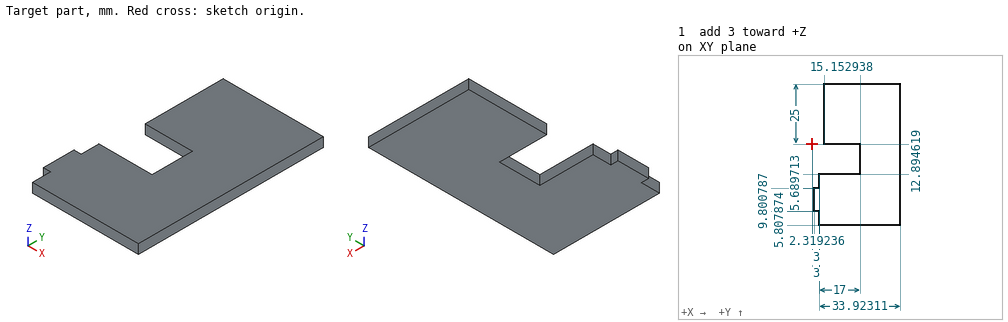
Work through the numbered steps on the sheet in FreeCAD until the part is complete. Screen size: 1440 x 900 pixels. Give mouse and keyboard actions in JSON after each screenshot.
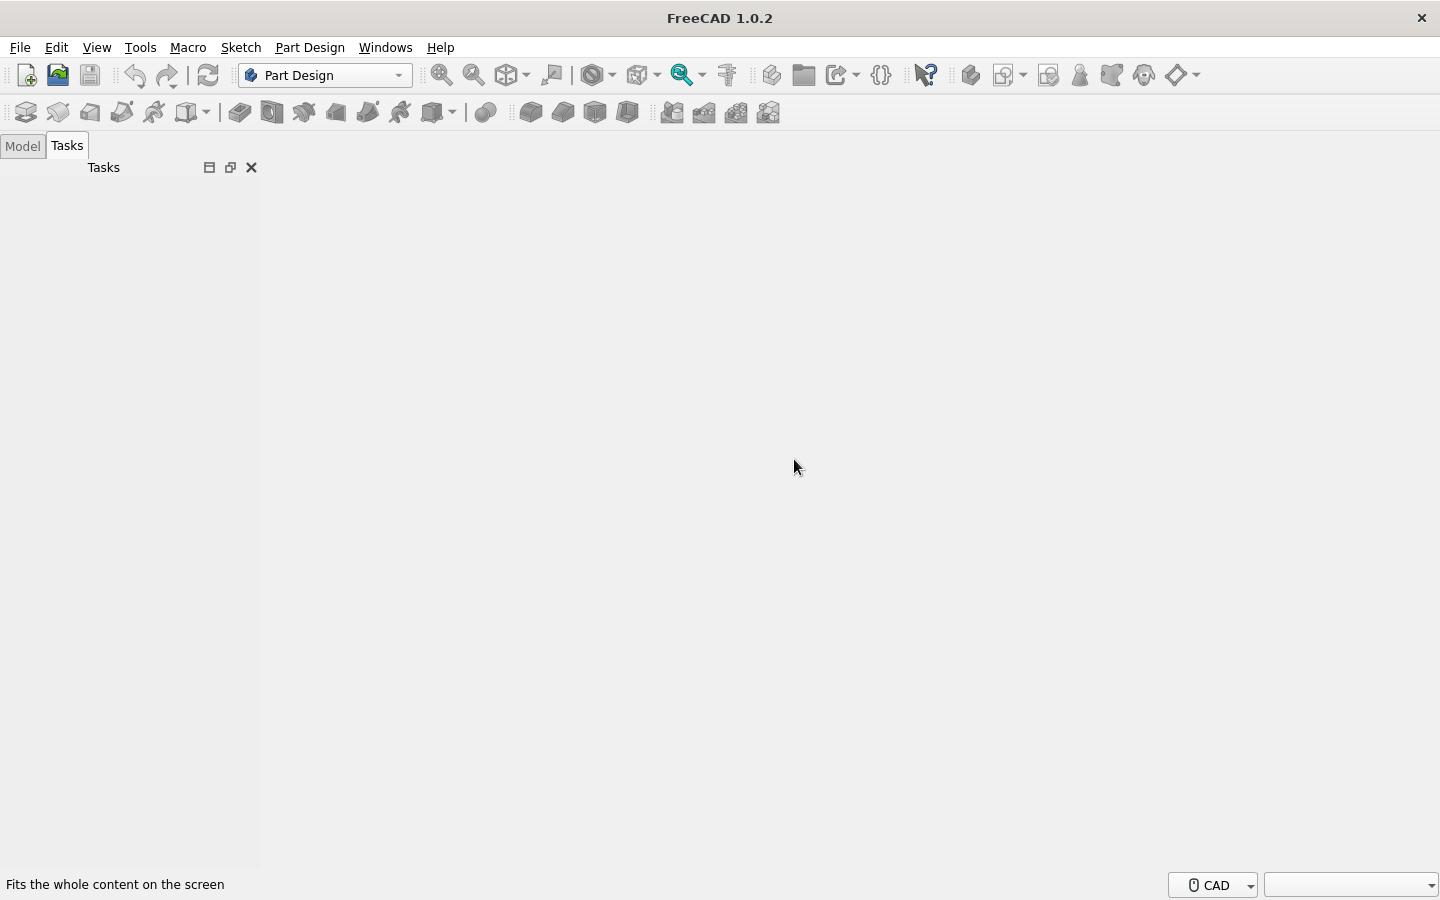
{"action": "left_click", "coordinate": [26, 76]}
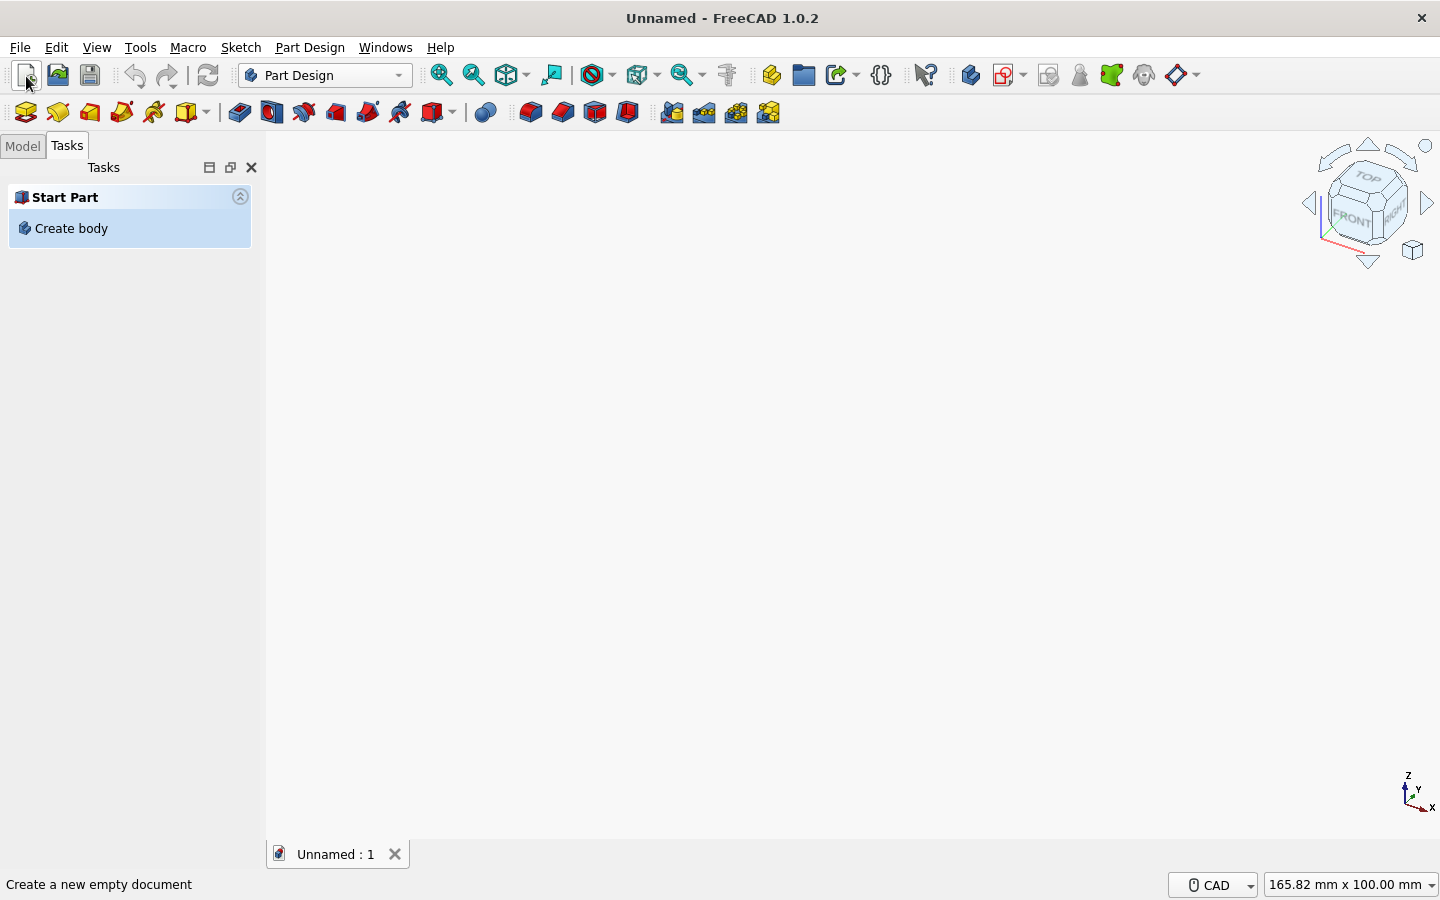
{"action": "left_click", "coordinate": [1004, 76]}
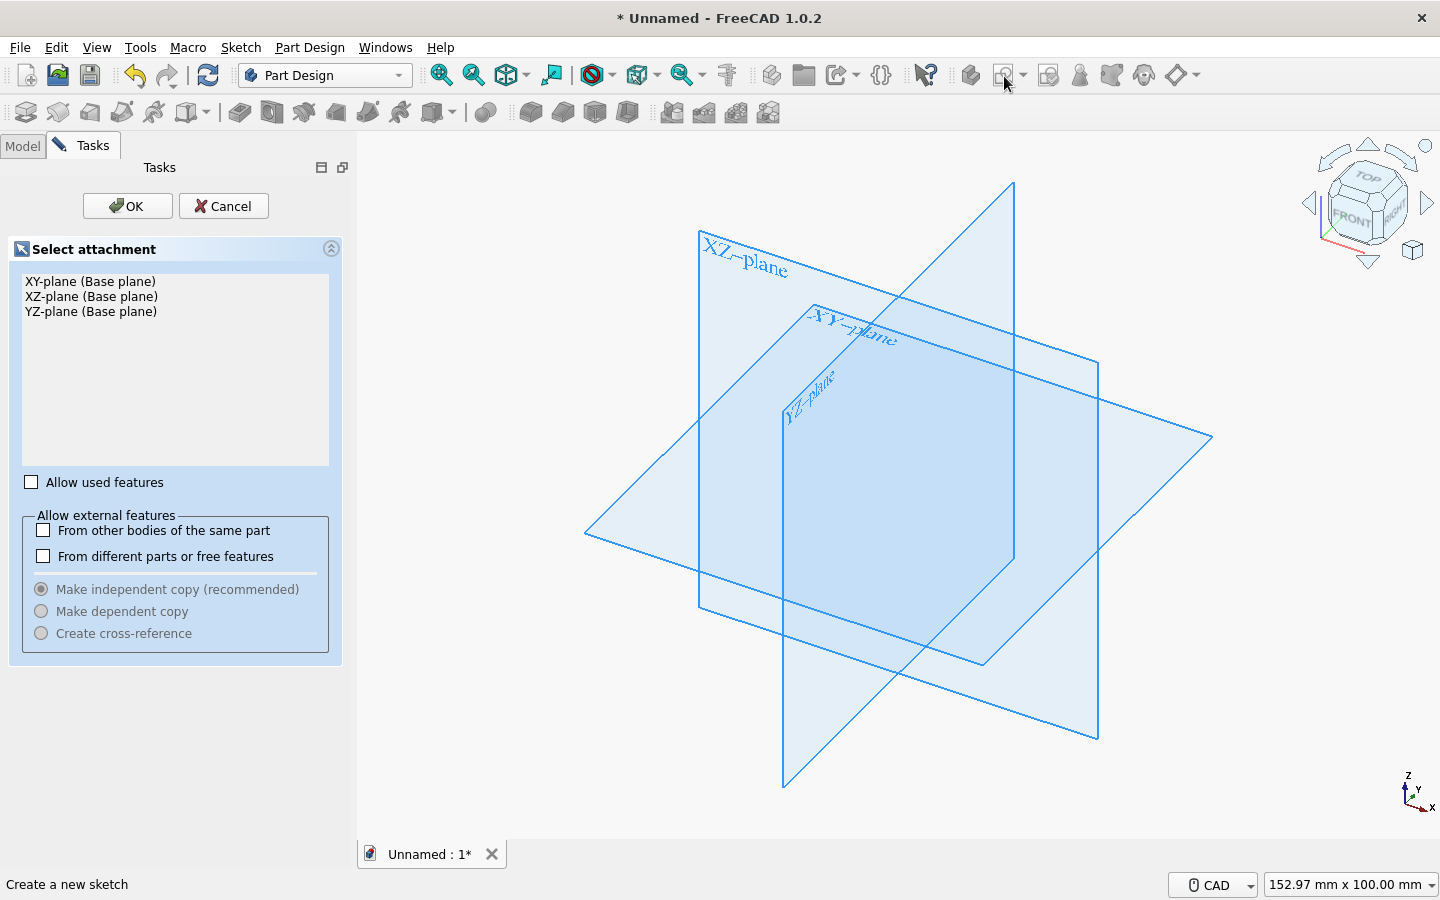
{"action": "left_click", "coordinate": [82, 282]}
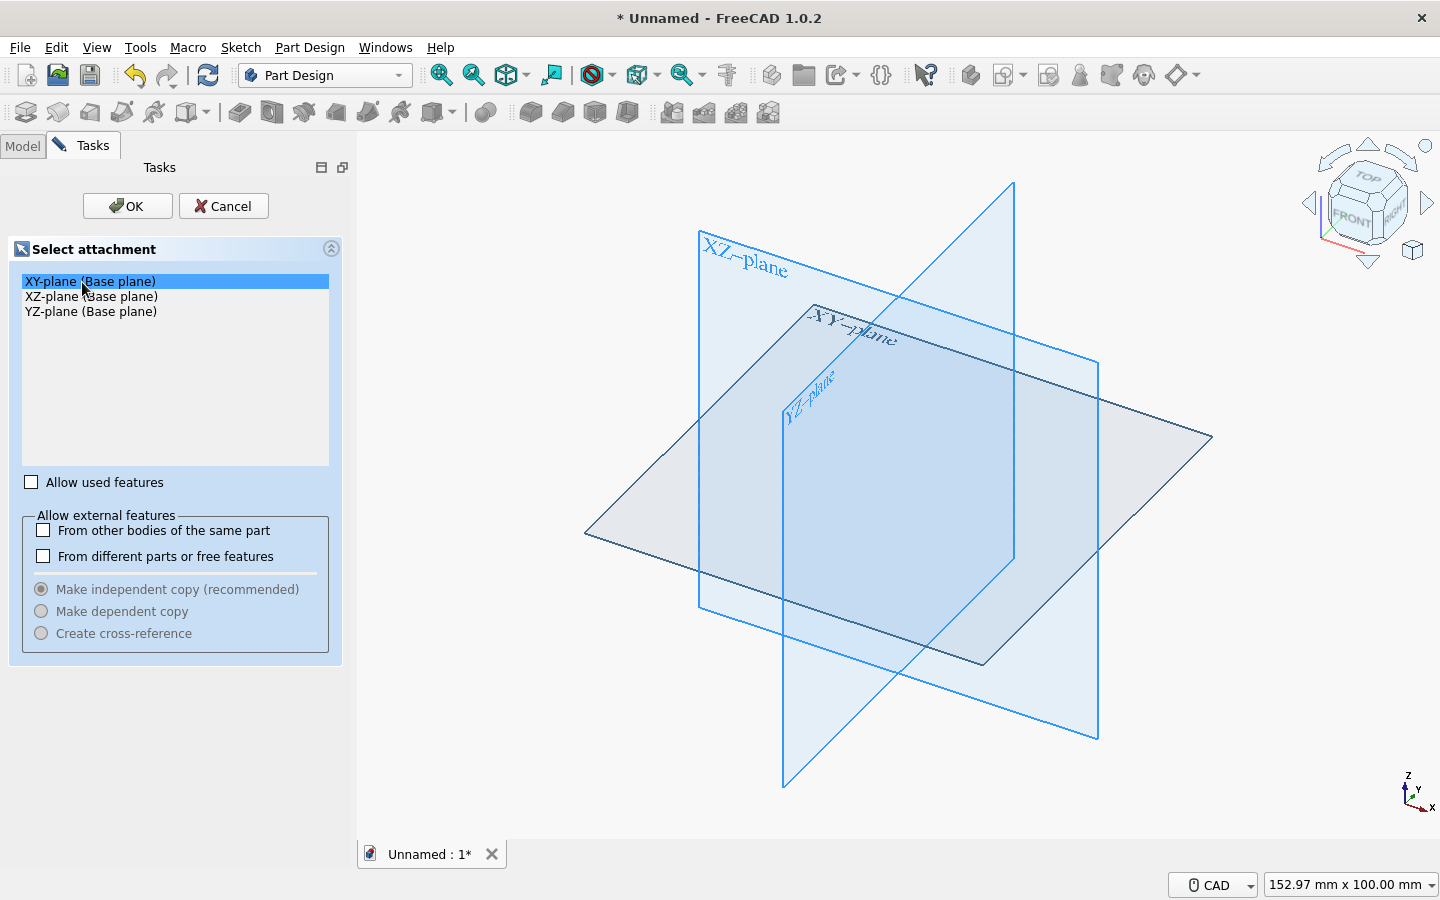
{"action": "left_click", "coordinate": [128, 206]}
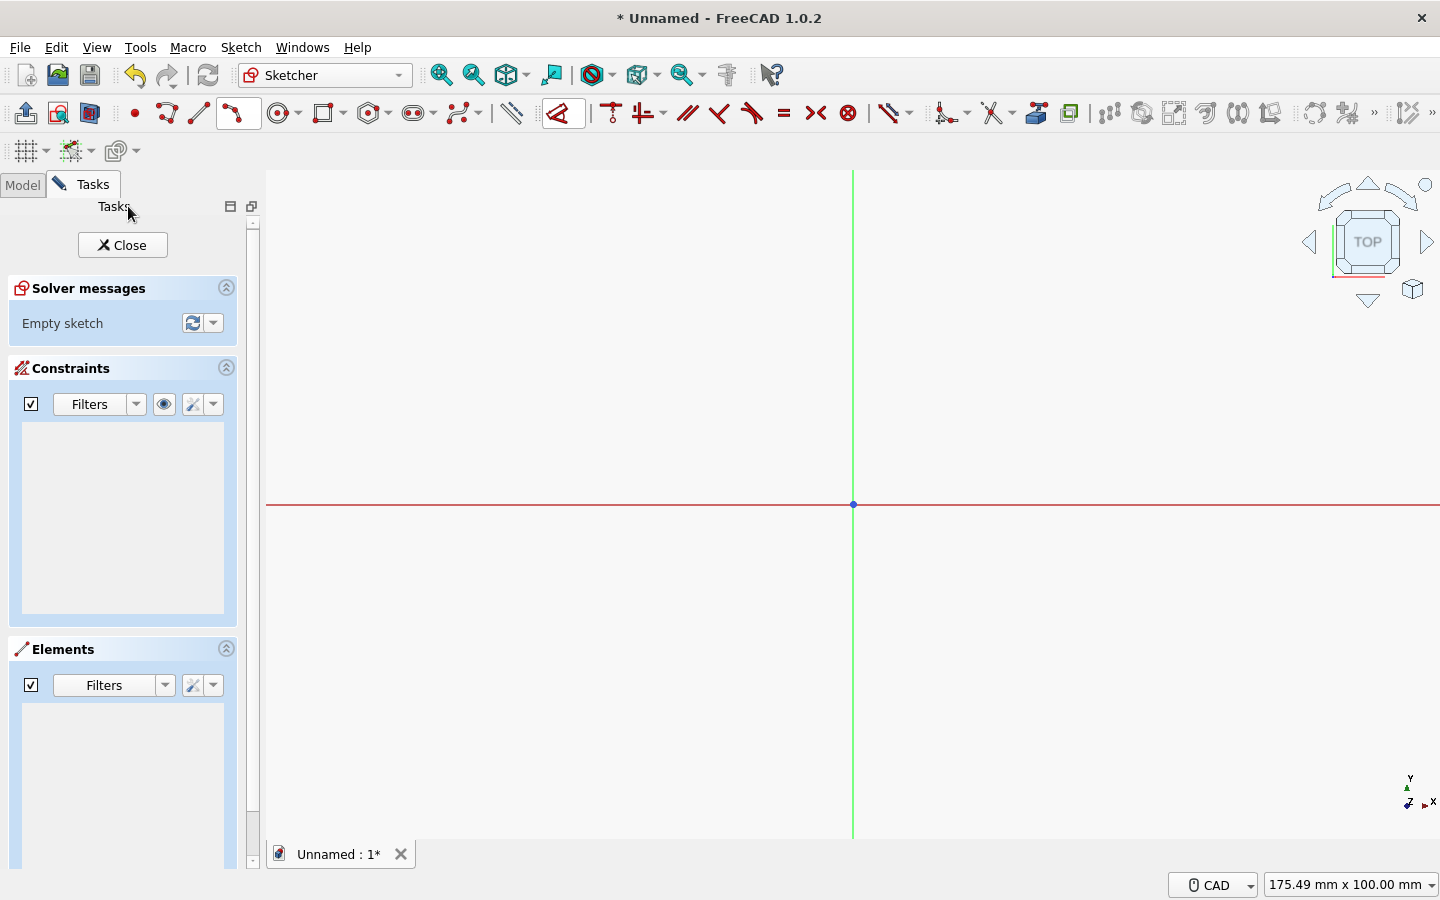
{"action": "left_click", "coordinate": [168, 114]}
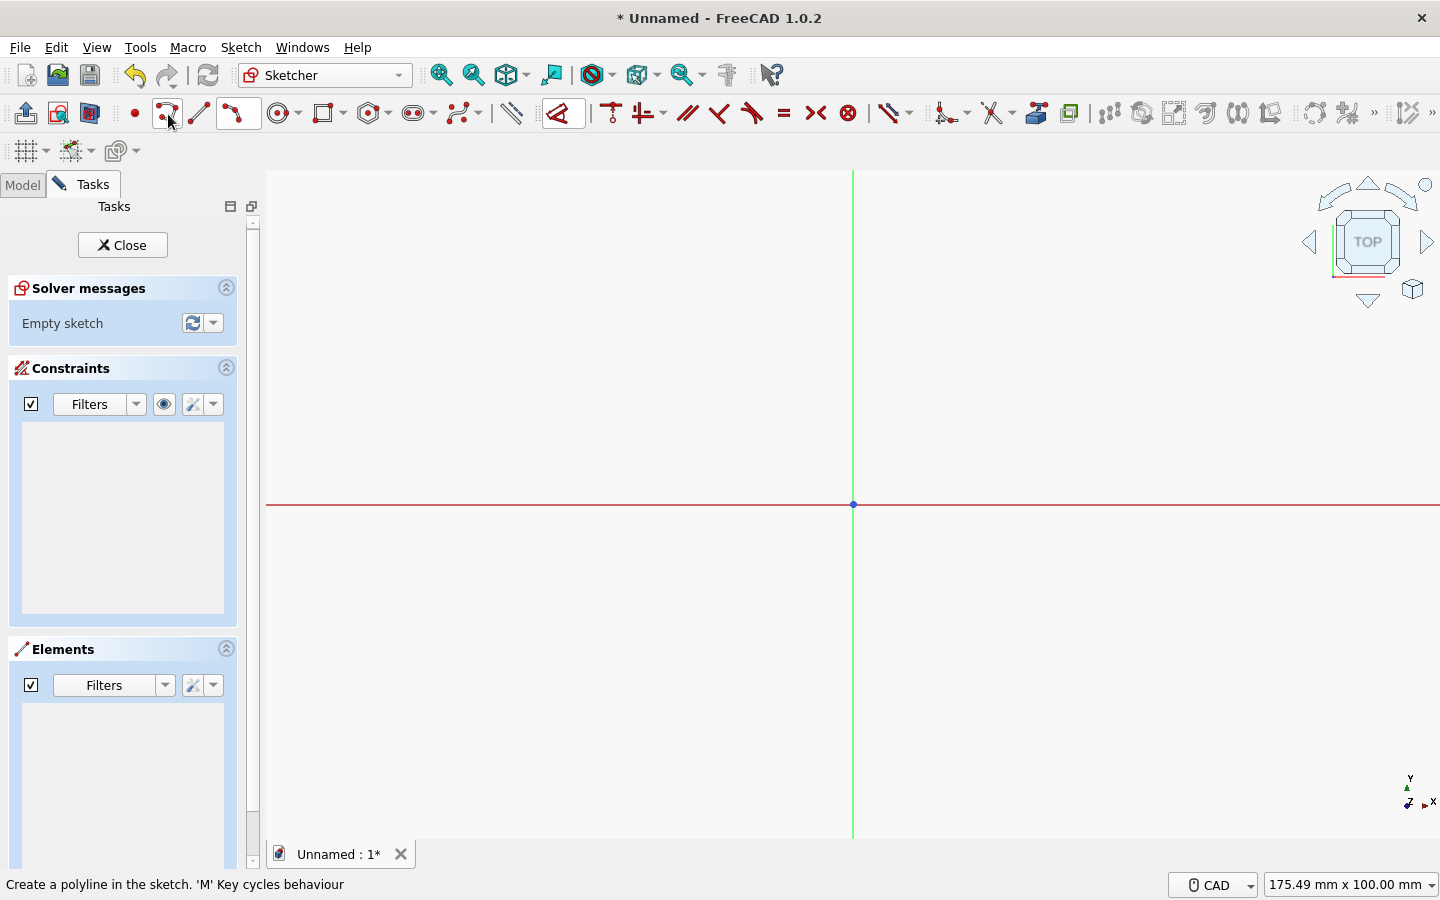
{"action": "left_click", "coordinate": [885, 504]}
{"action": "left_click", "coordinate": [987, 514]}
{"action": "left_click", "coordinate": [987, 591]}
{"action": "left_click", "coordinate": [873, 591]}
{"action": "left_click", "coordinate": [873, 629]}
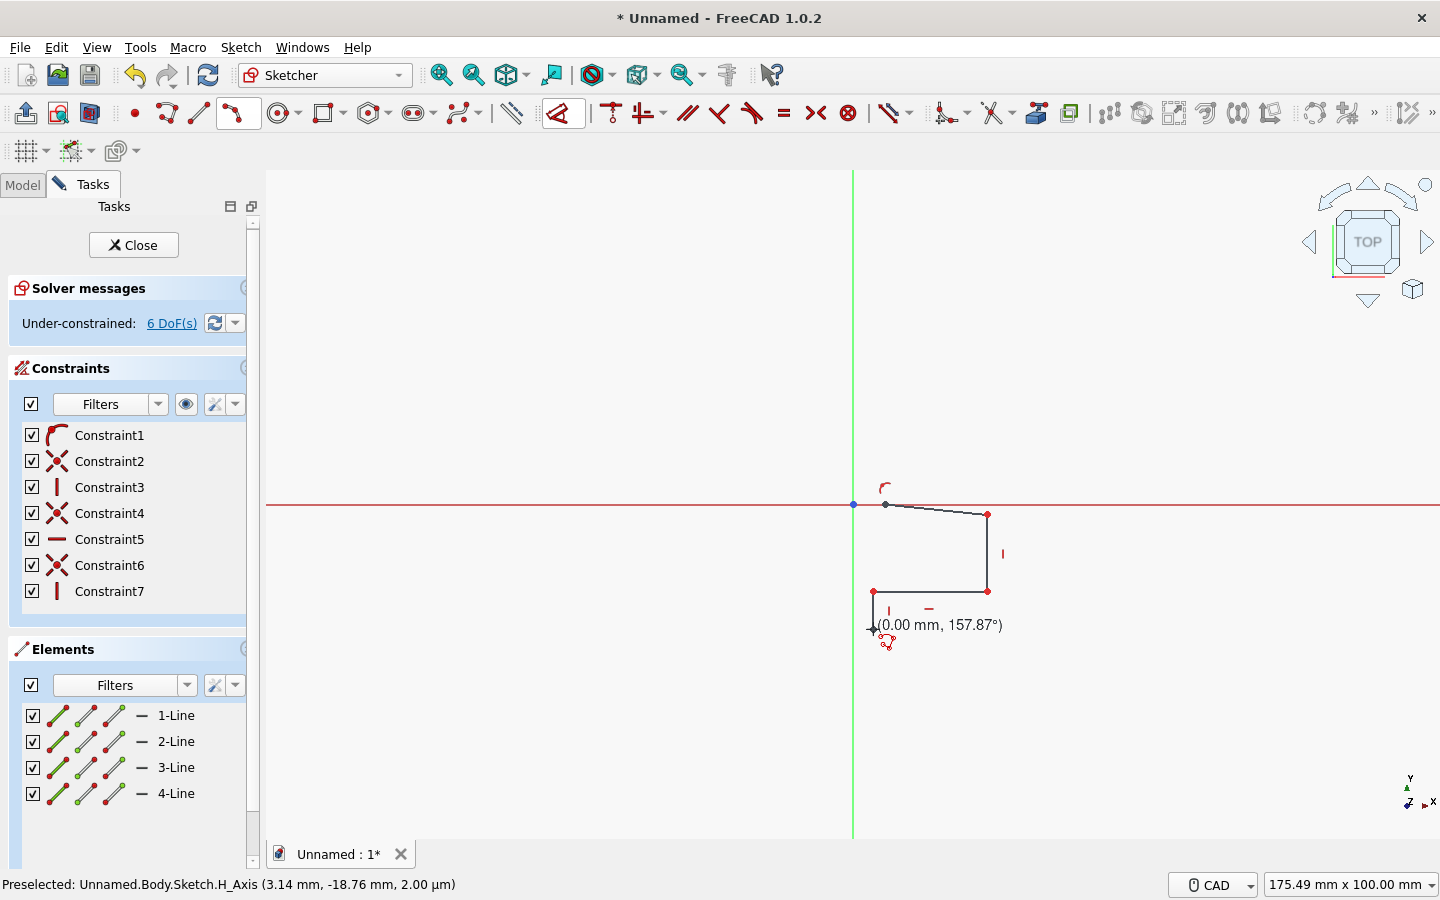
{"action": "scroll", "coordinate": [858, 629], "scroll_direction": "up", "scroll_amount": 7}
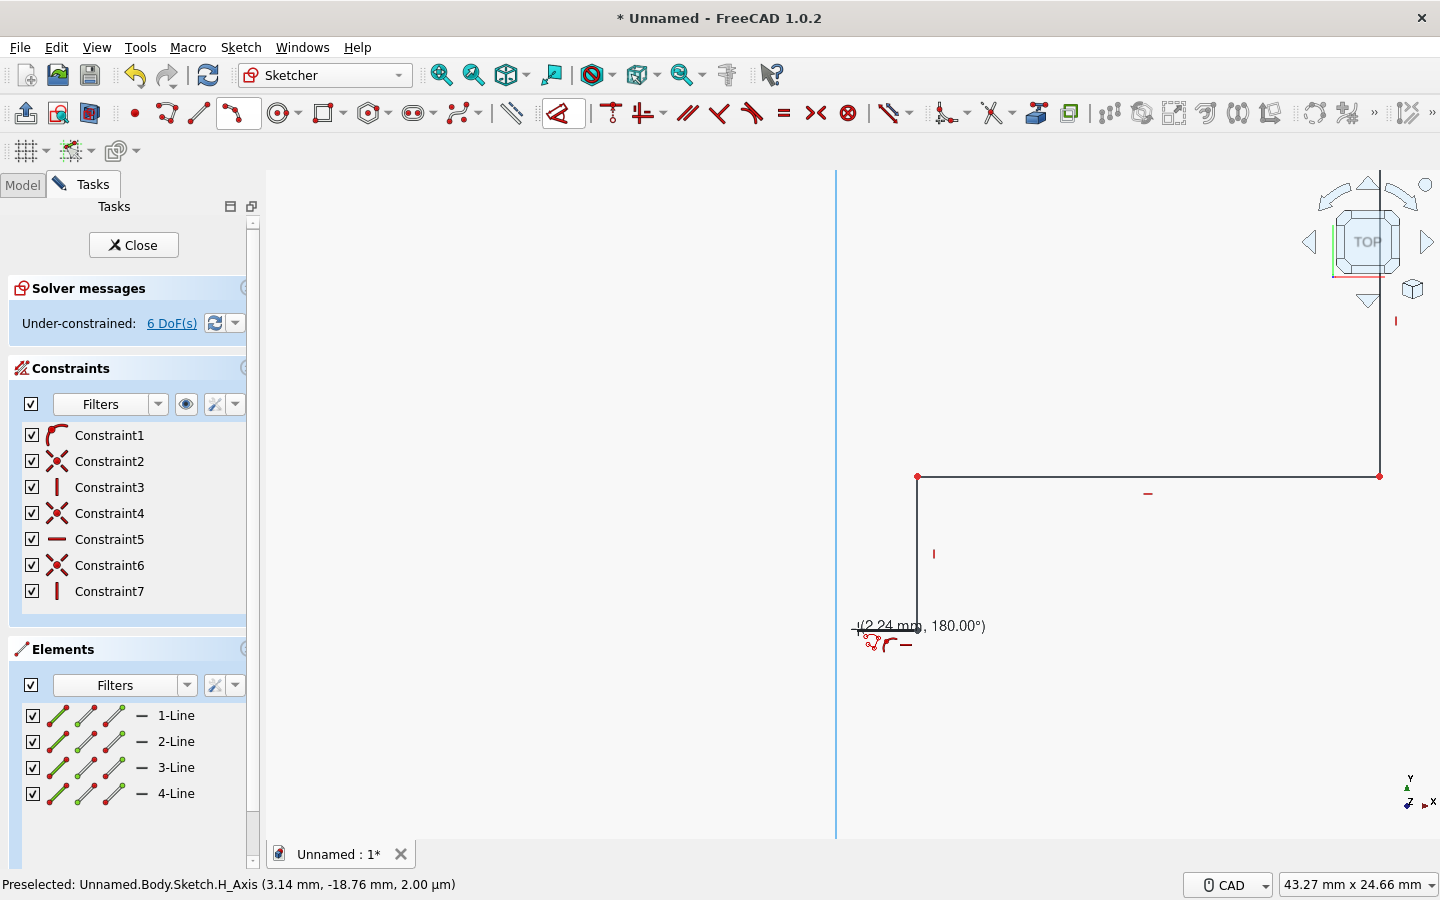
{"action": "left_click", "coordinate": [855, 627]}